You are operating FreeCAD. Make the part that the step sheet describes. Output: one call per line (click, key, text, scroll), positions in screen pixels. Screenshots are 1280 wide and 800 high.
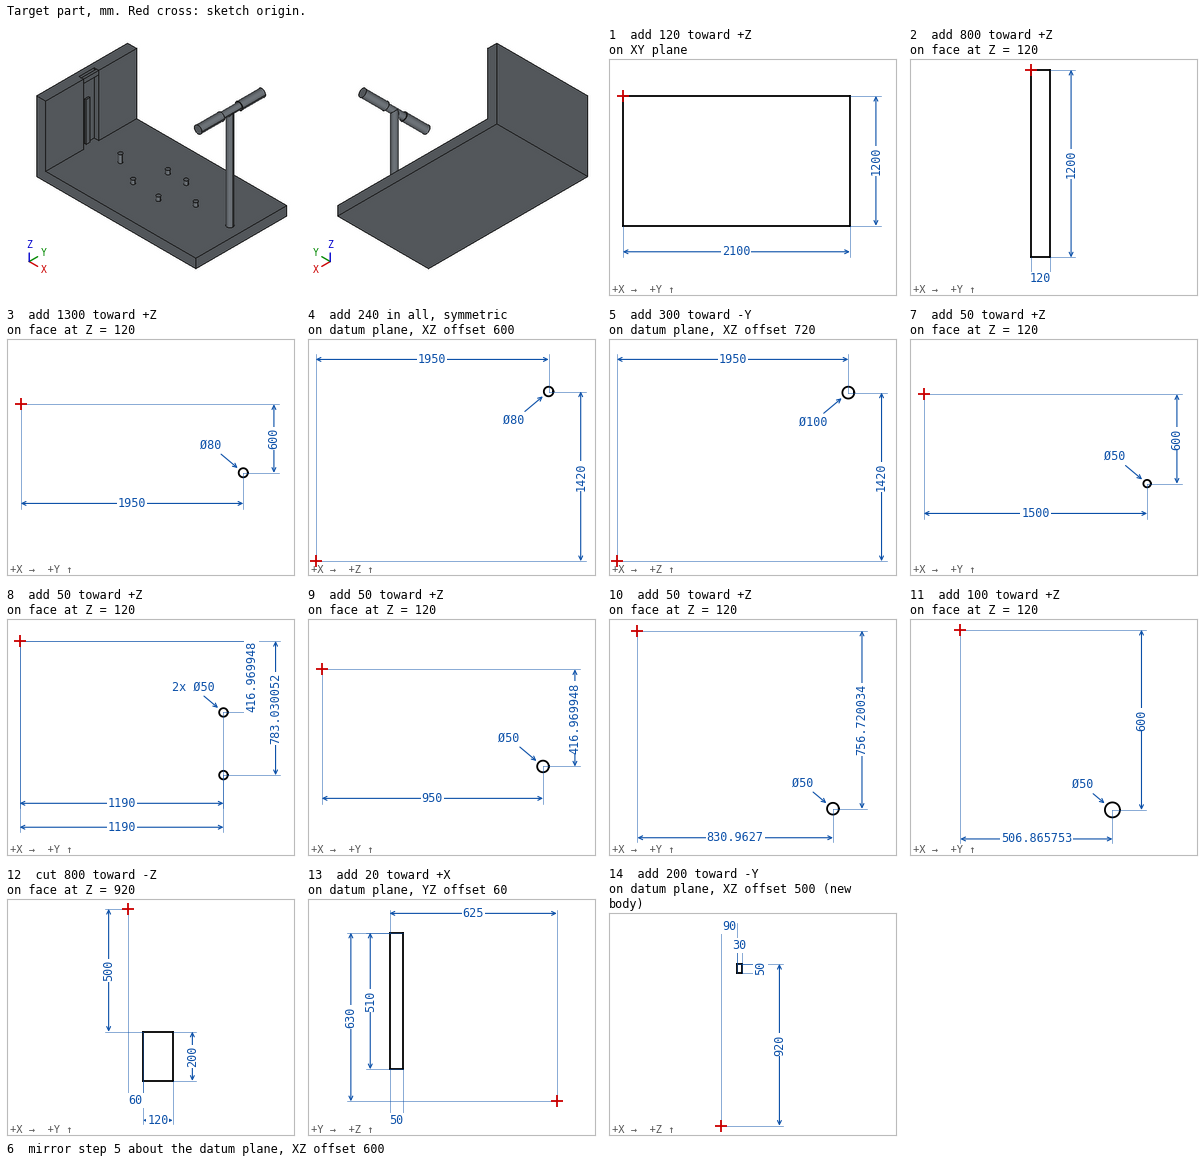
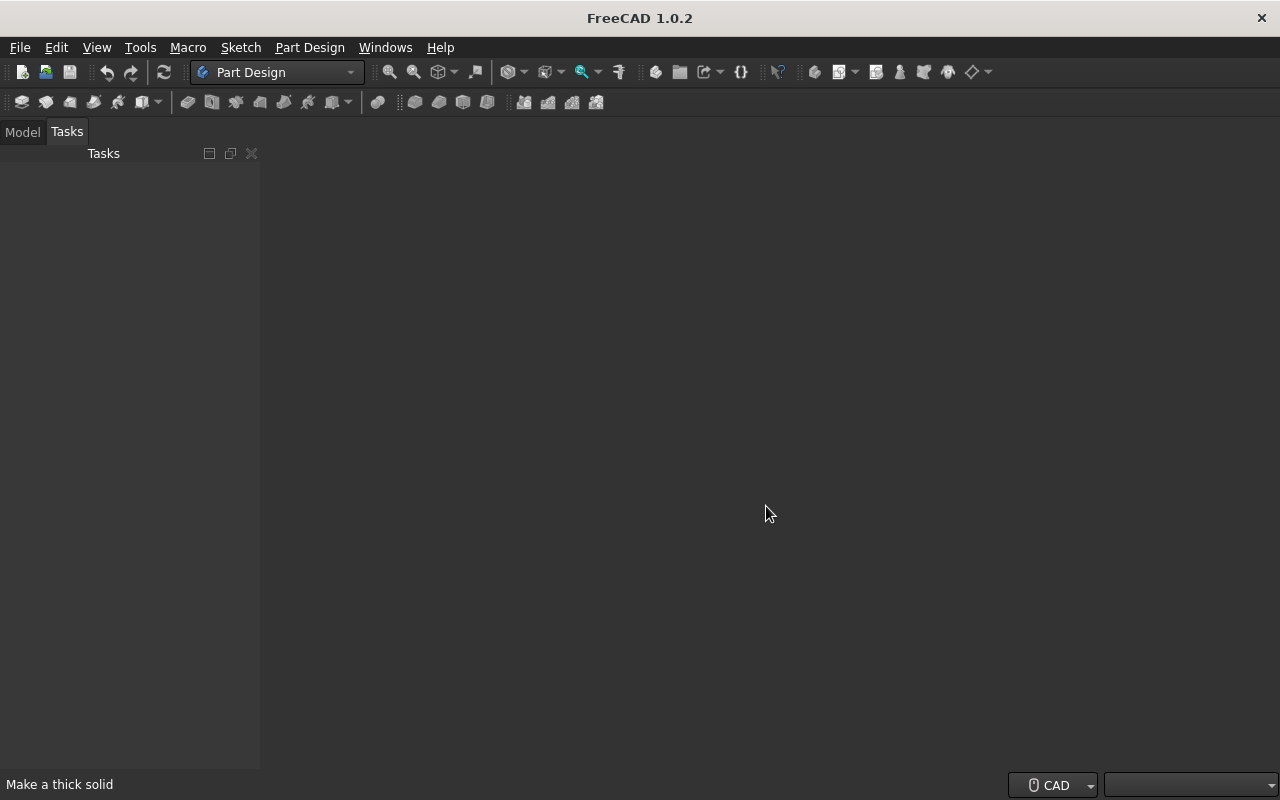
click(22, 72)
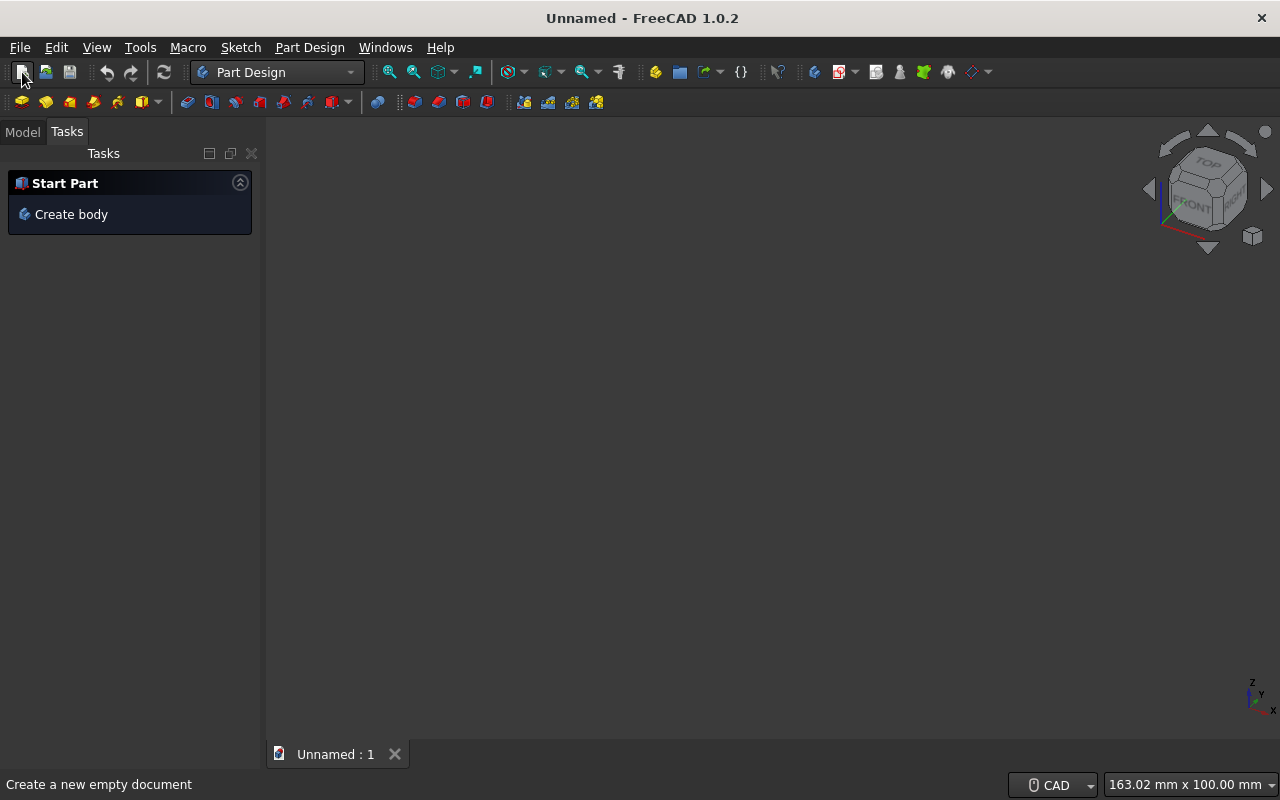
click(840, 72)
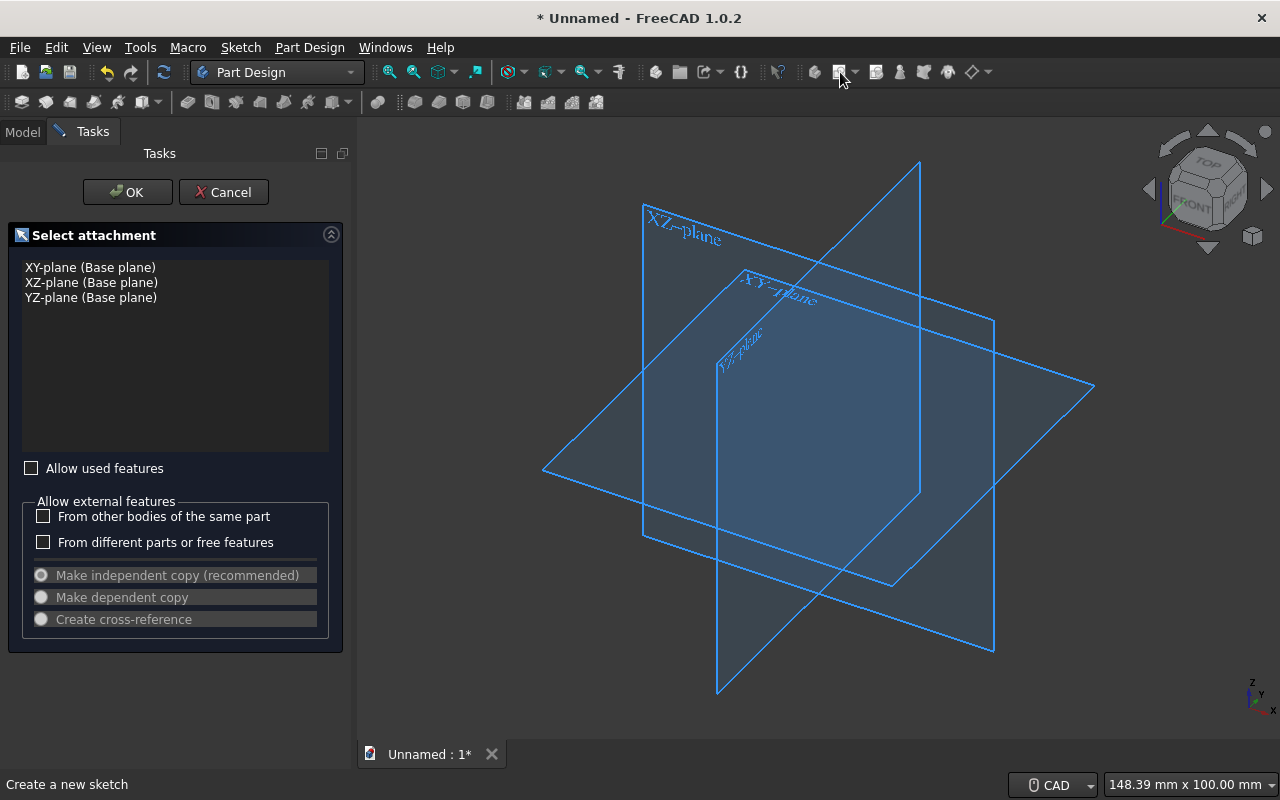
click(82, 268)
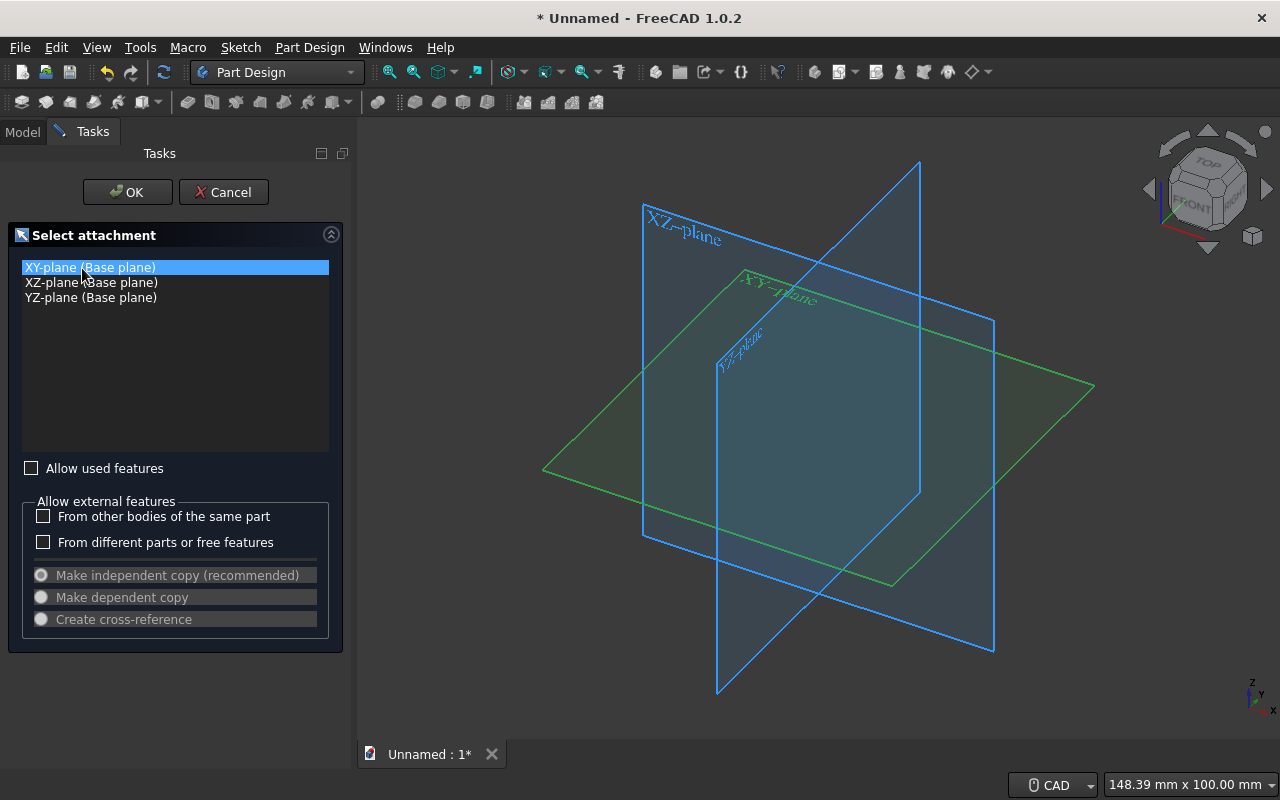
click(128, 192)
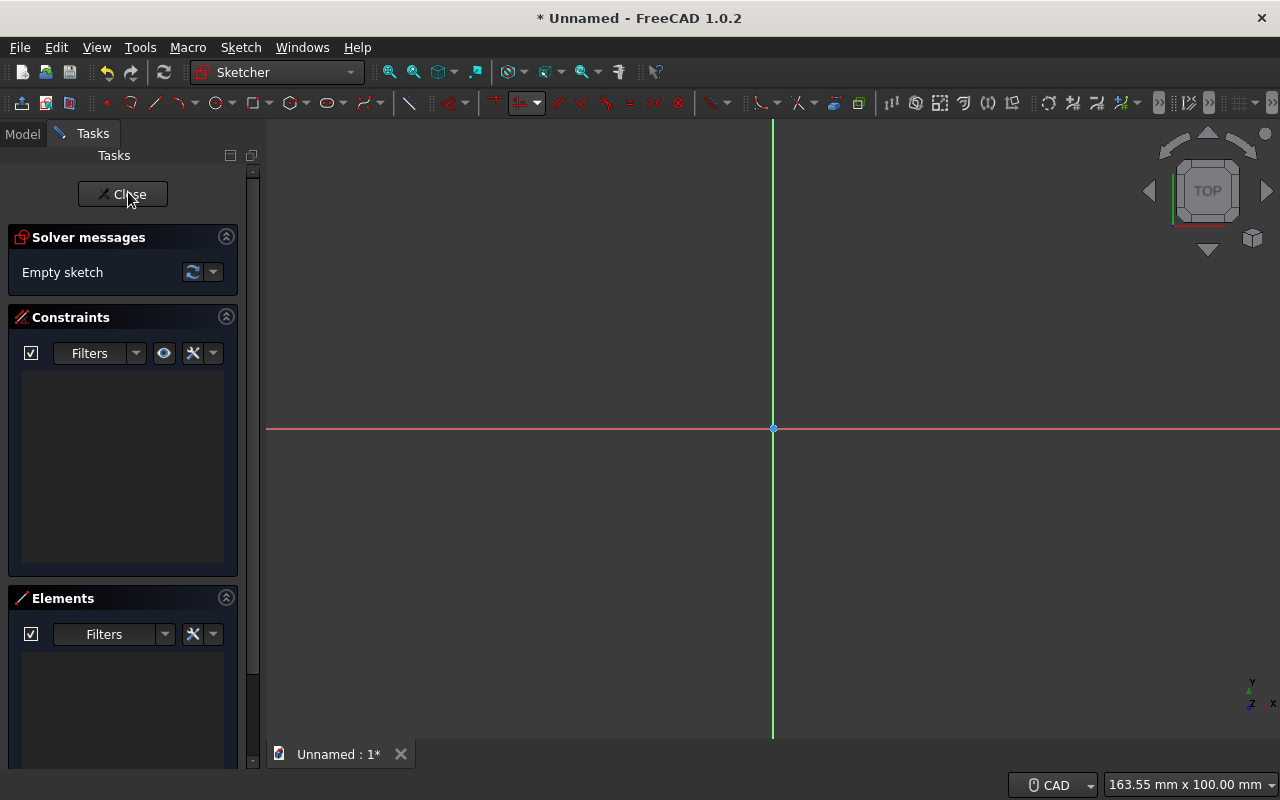
scroll(360, 234, down, 15)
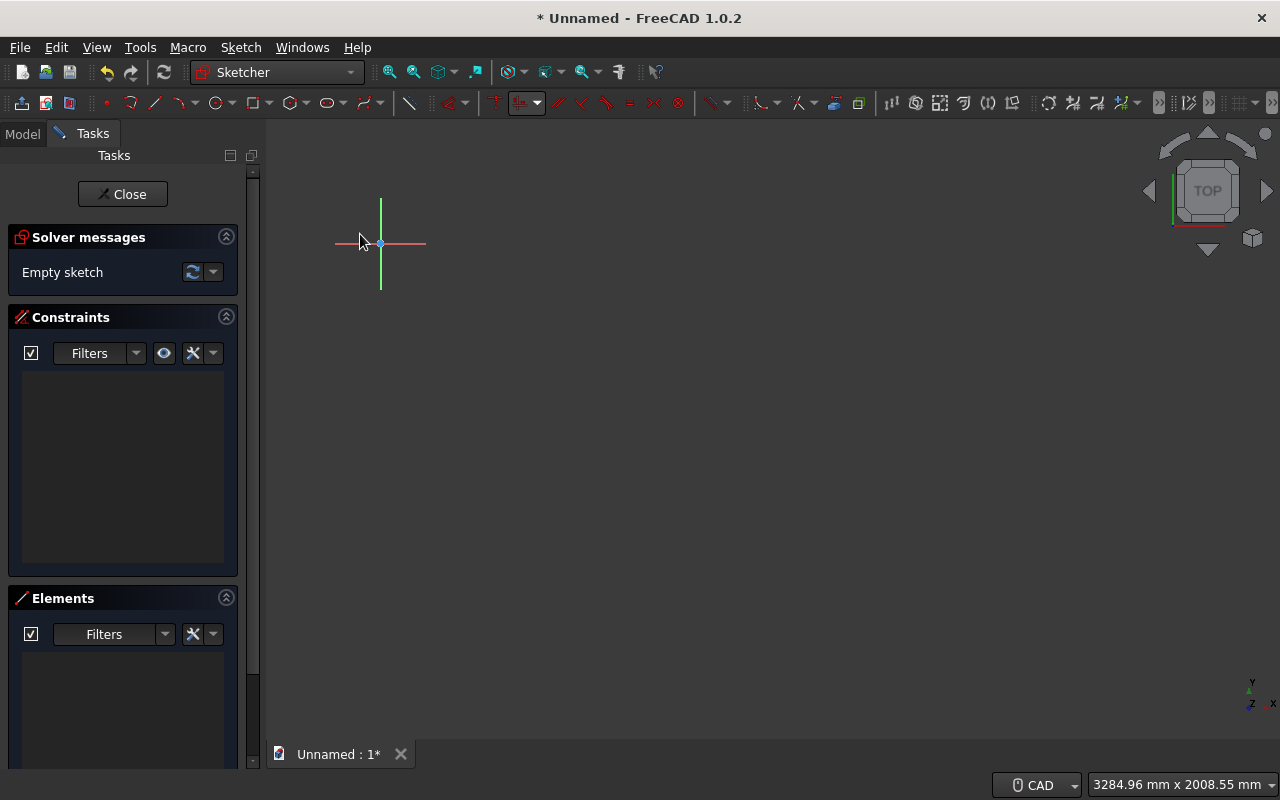
click(254, 104)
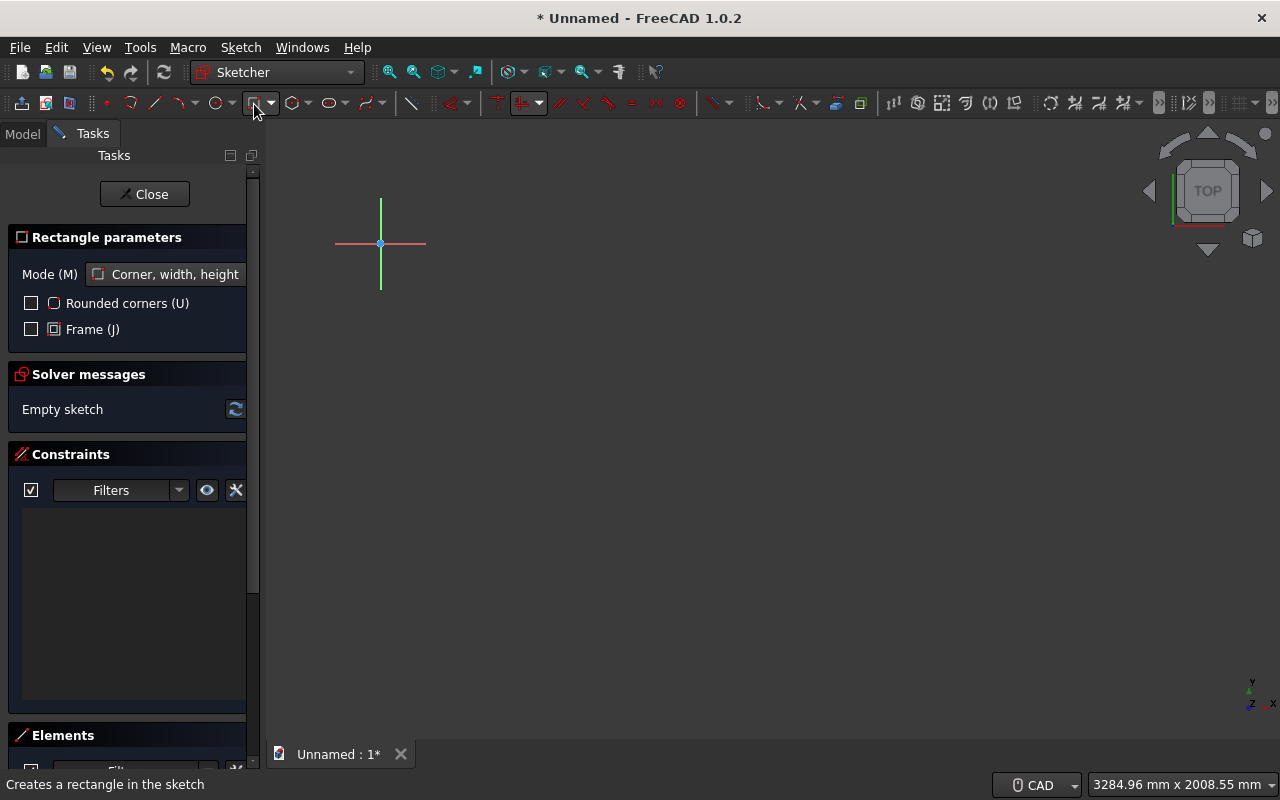
click(381, 244)
move(1029, 614)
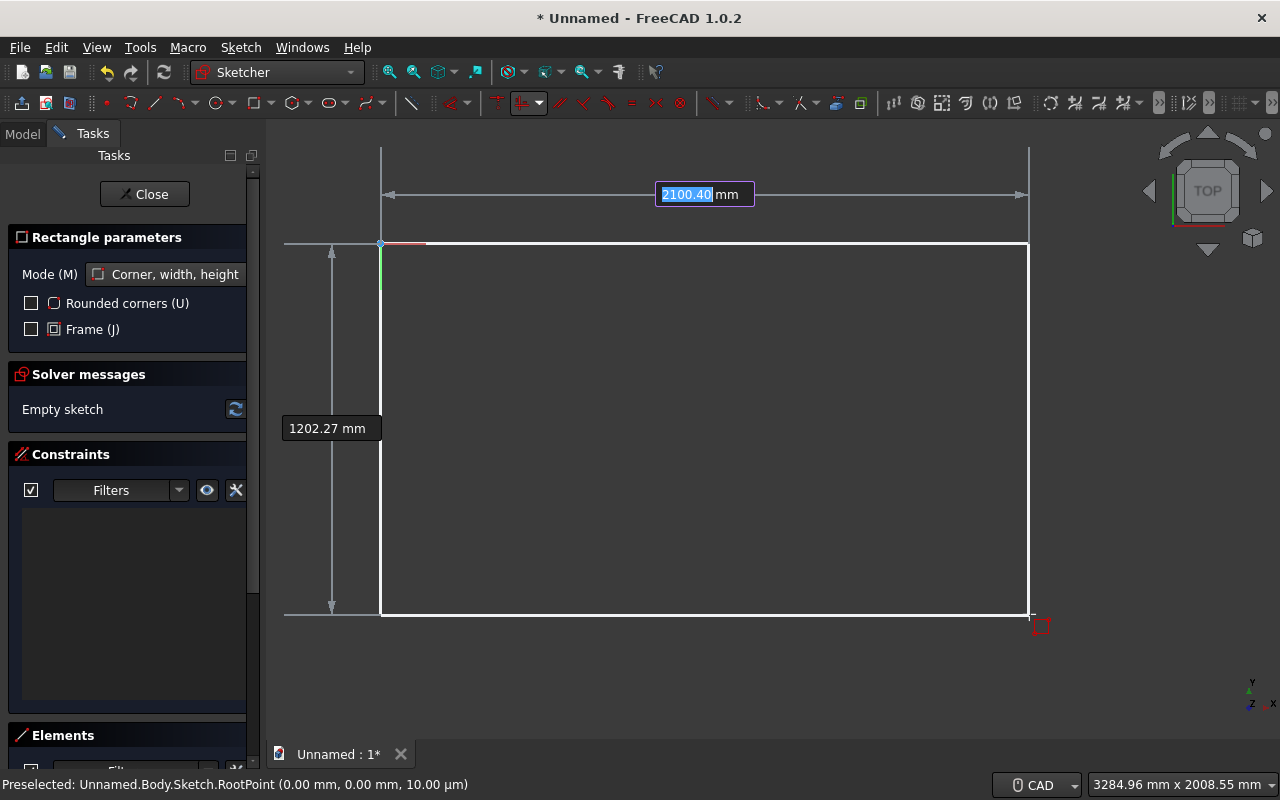
text(2100)
key(Tab)
text(1200)
key(Return)
key(Escape)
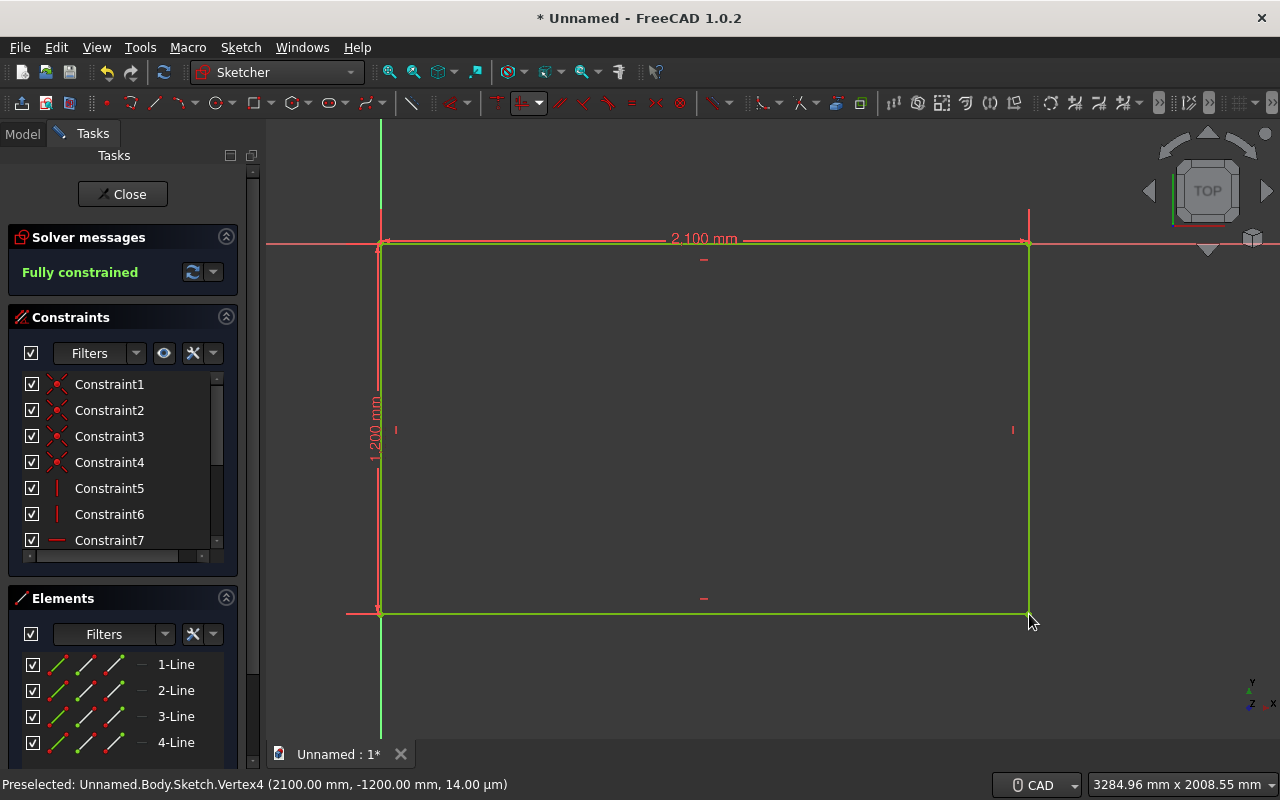
click(123, 194)